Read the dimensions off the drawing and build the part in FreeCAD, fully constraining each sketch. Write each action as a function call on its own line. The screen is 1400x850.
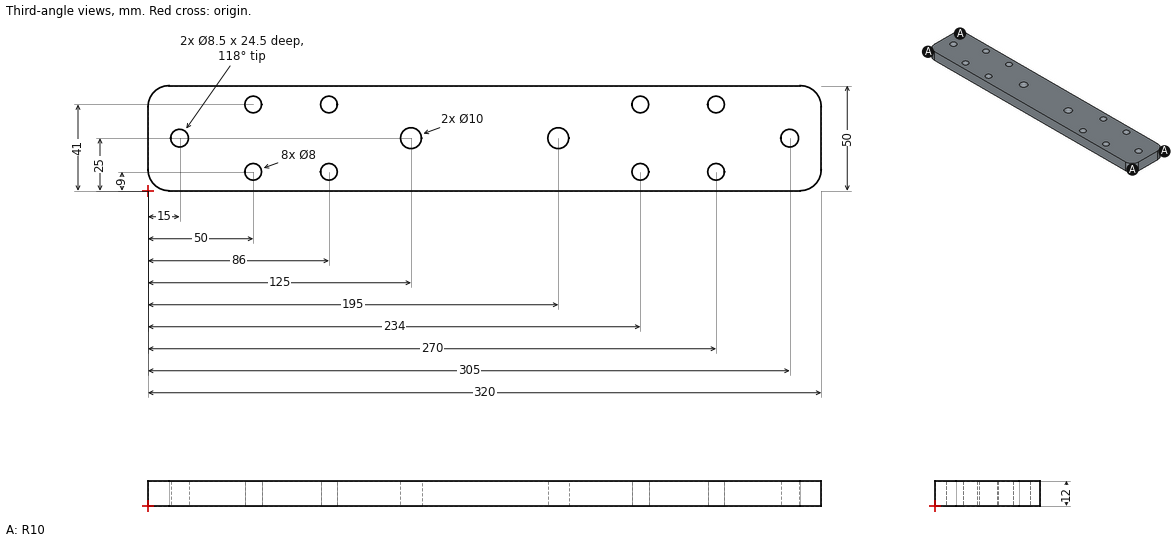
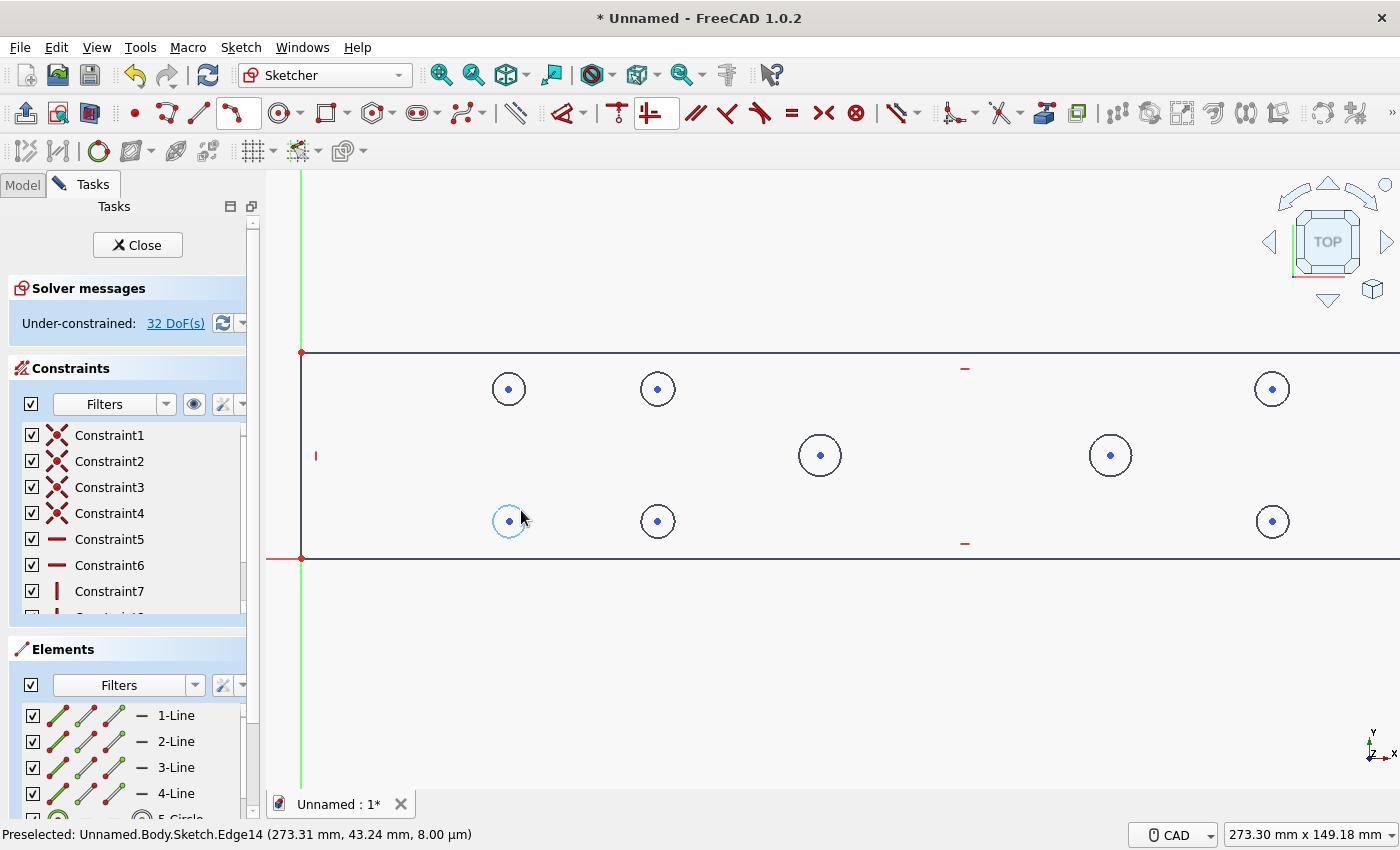
click(521, 510)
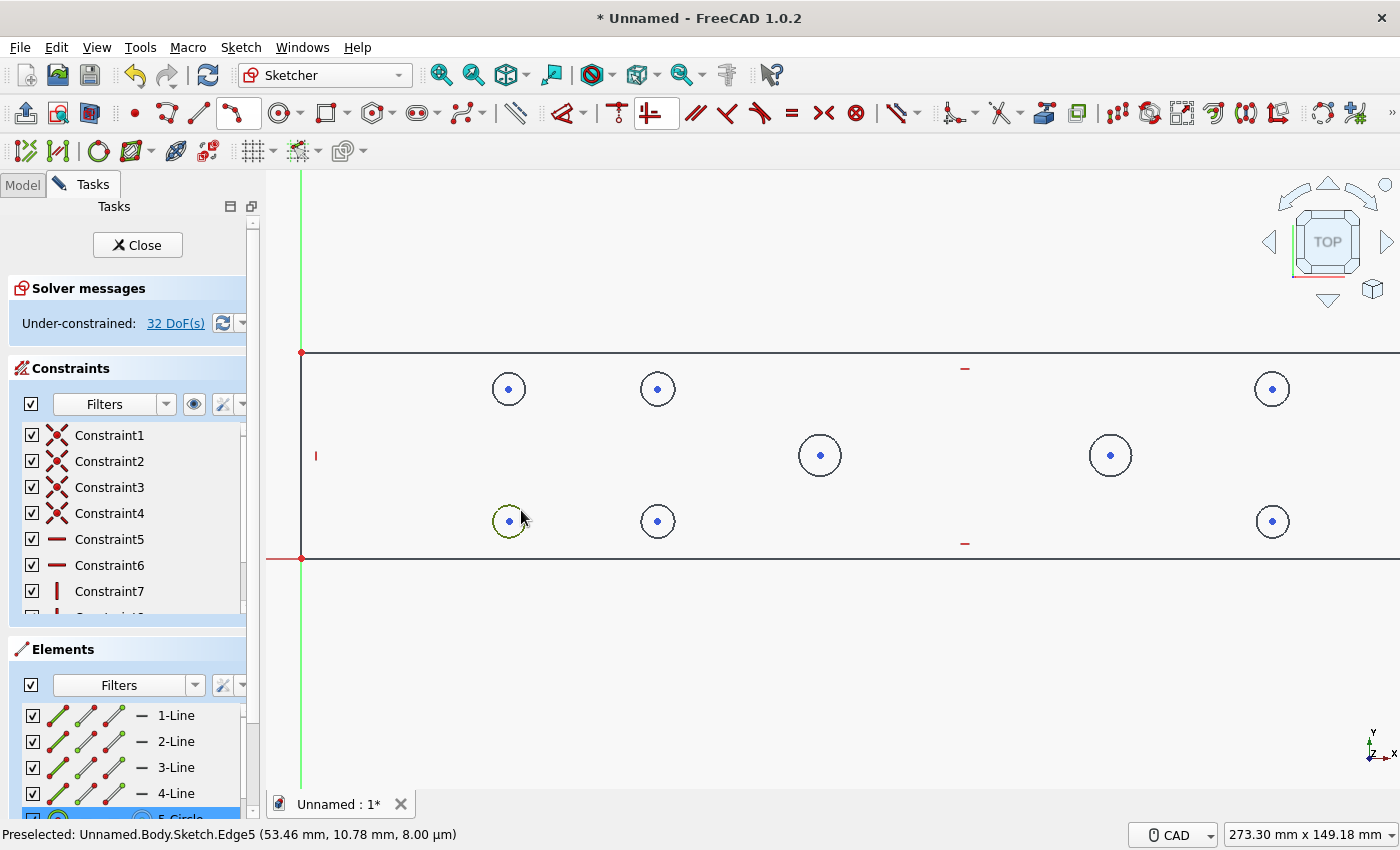
click(670, 510)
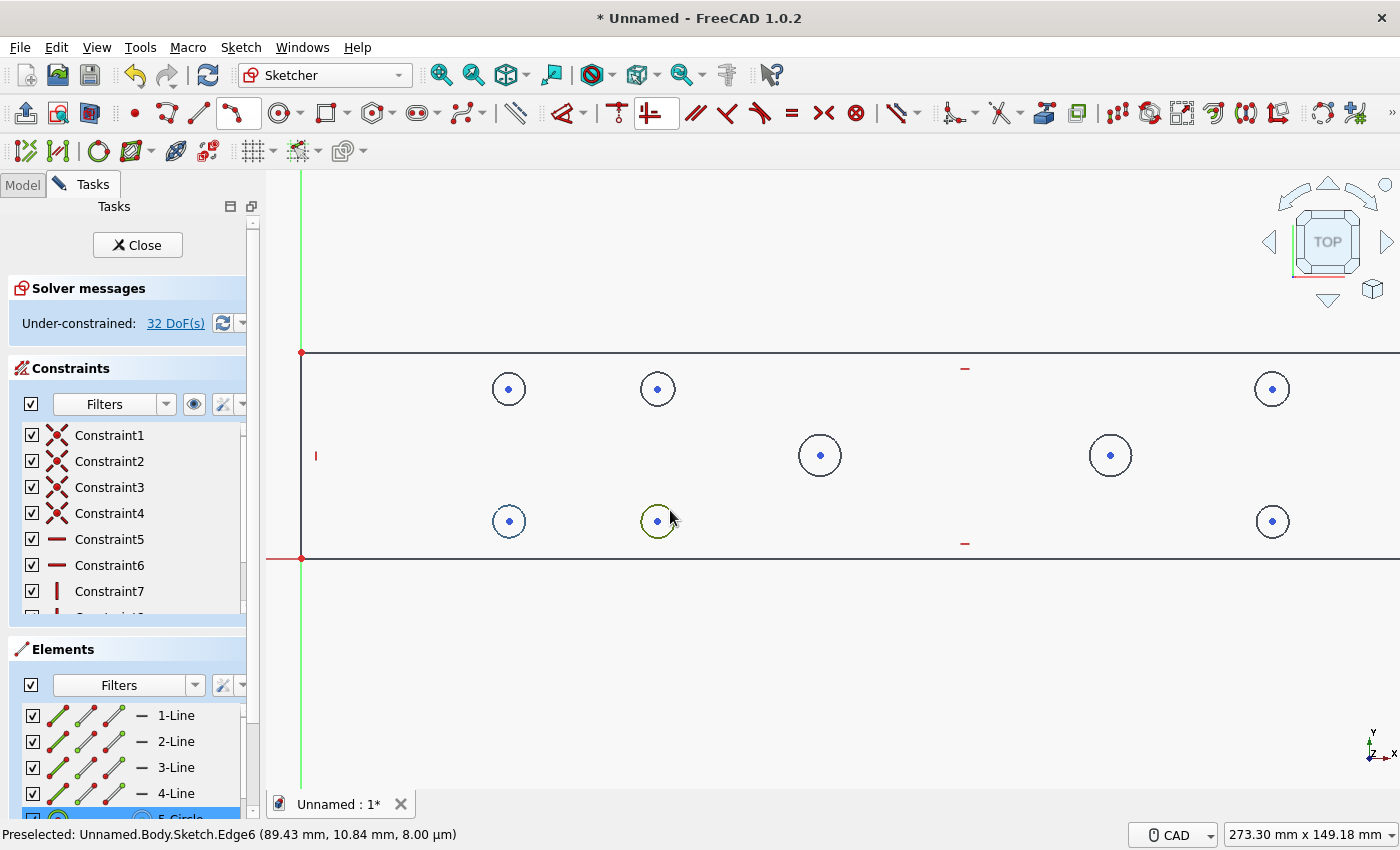
scroll(520, 510, down, 3)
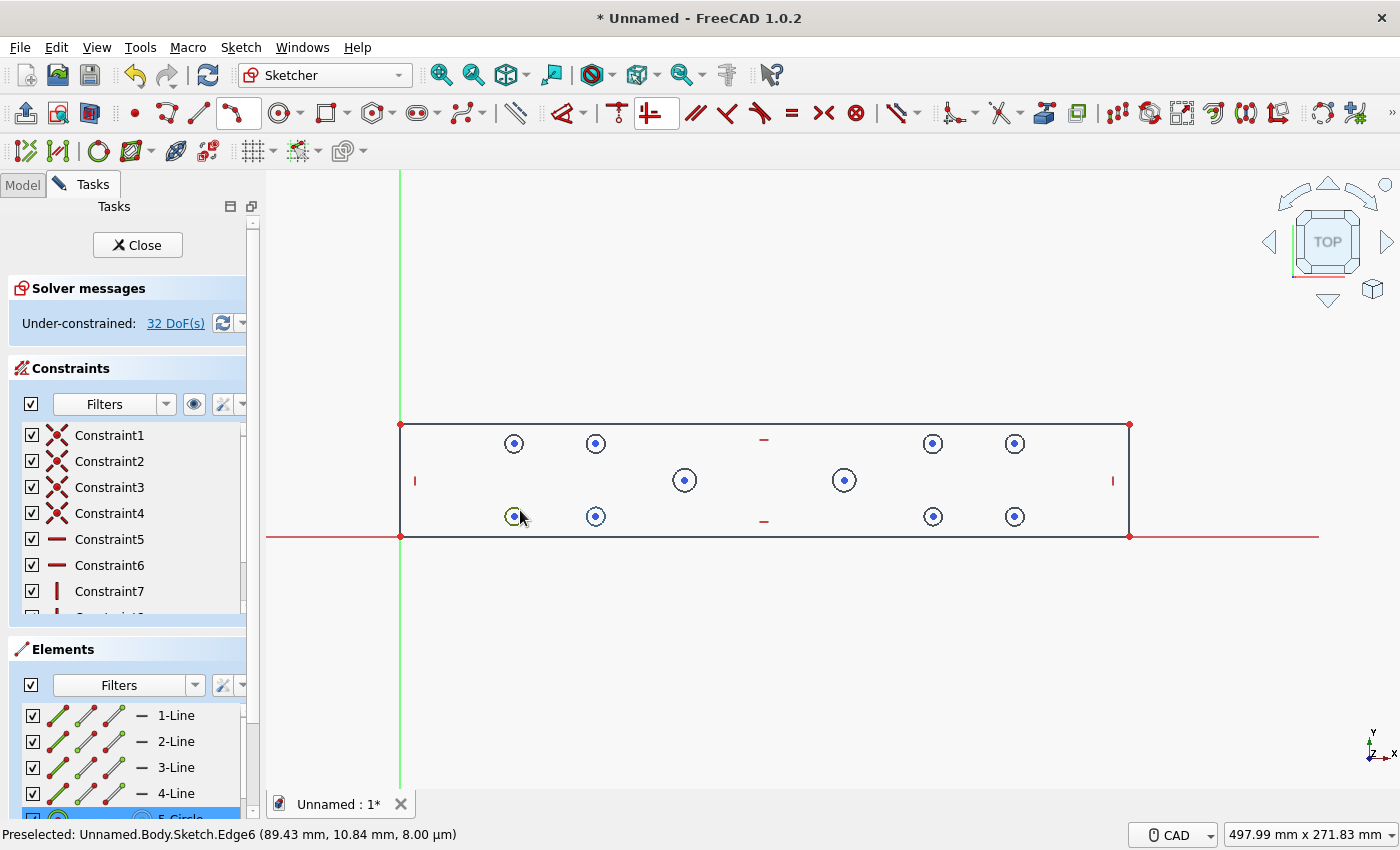
scroll(939, 510, up, 3)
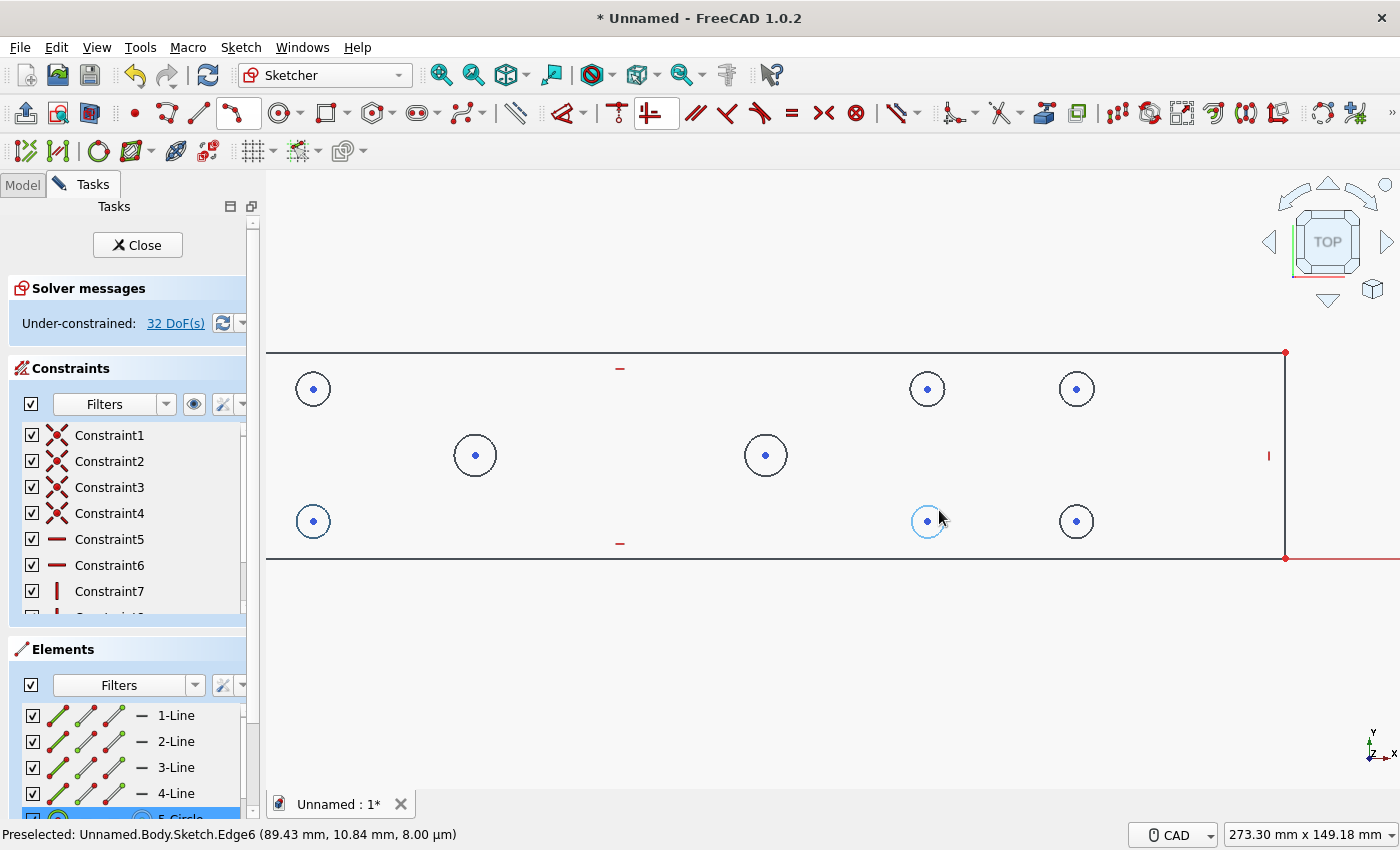
click(939, 510)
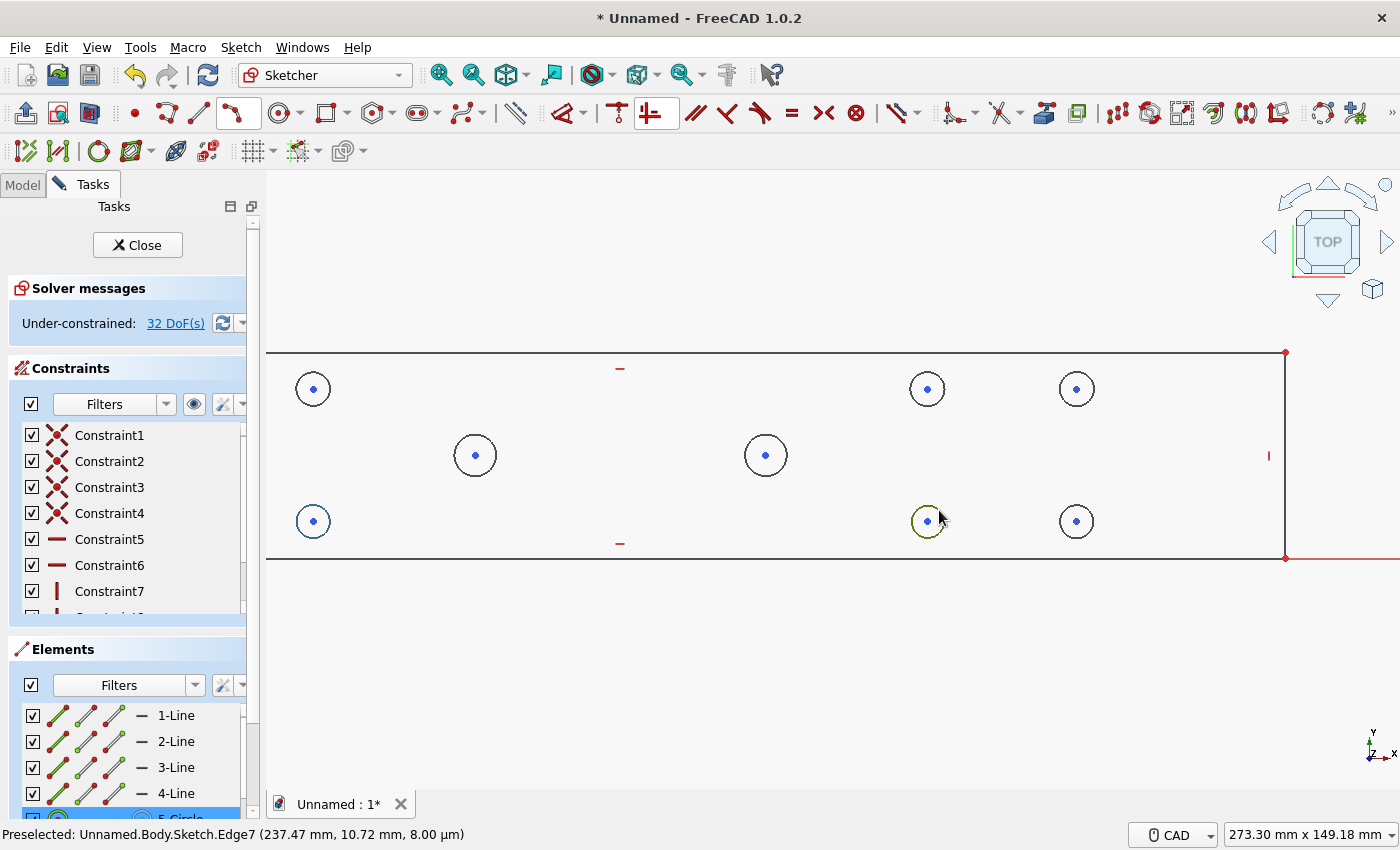
click(1088, 510)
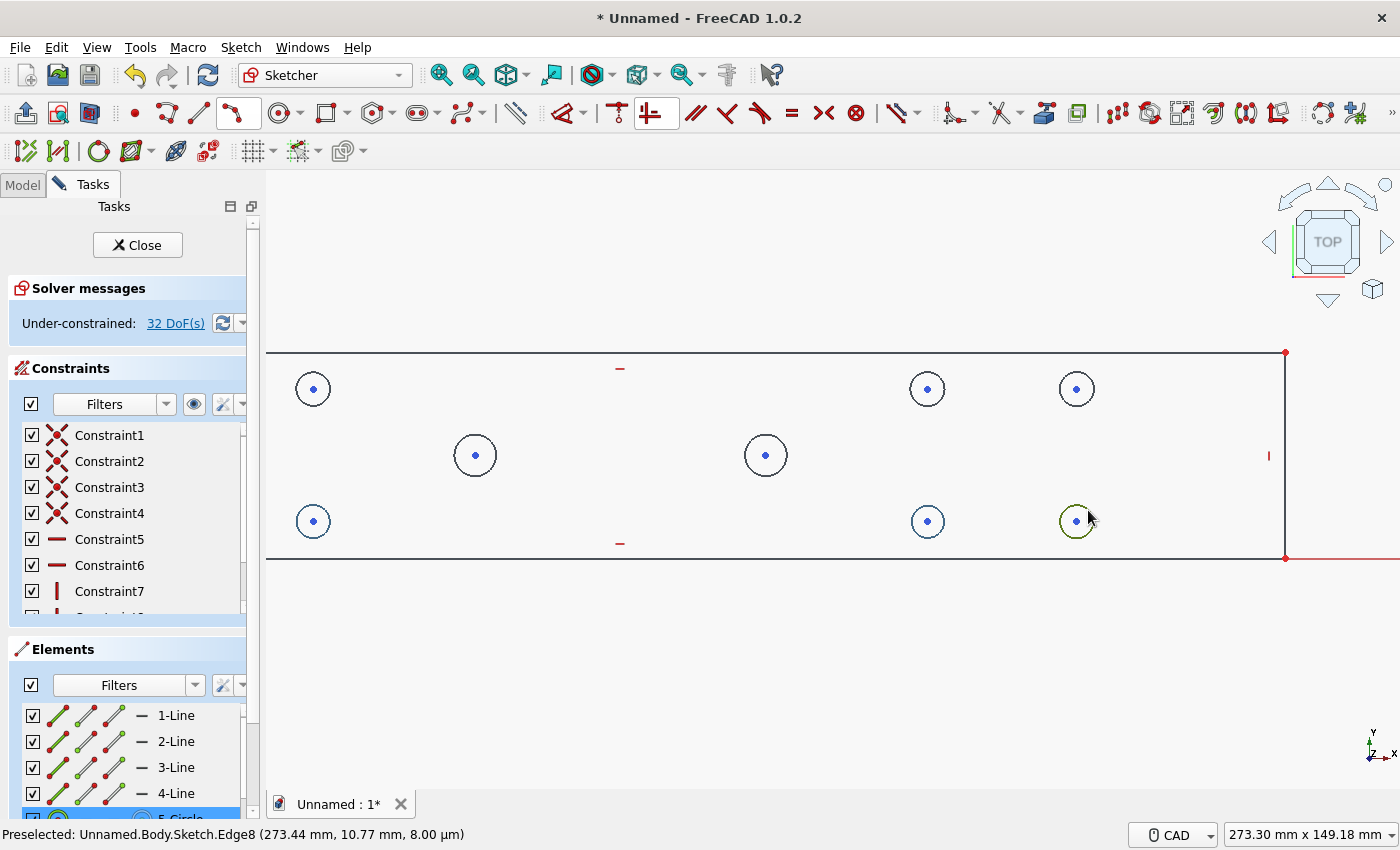
scroll(940, 510, down, 3)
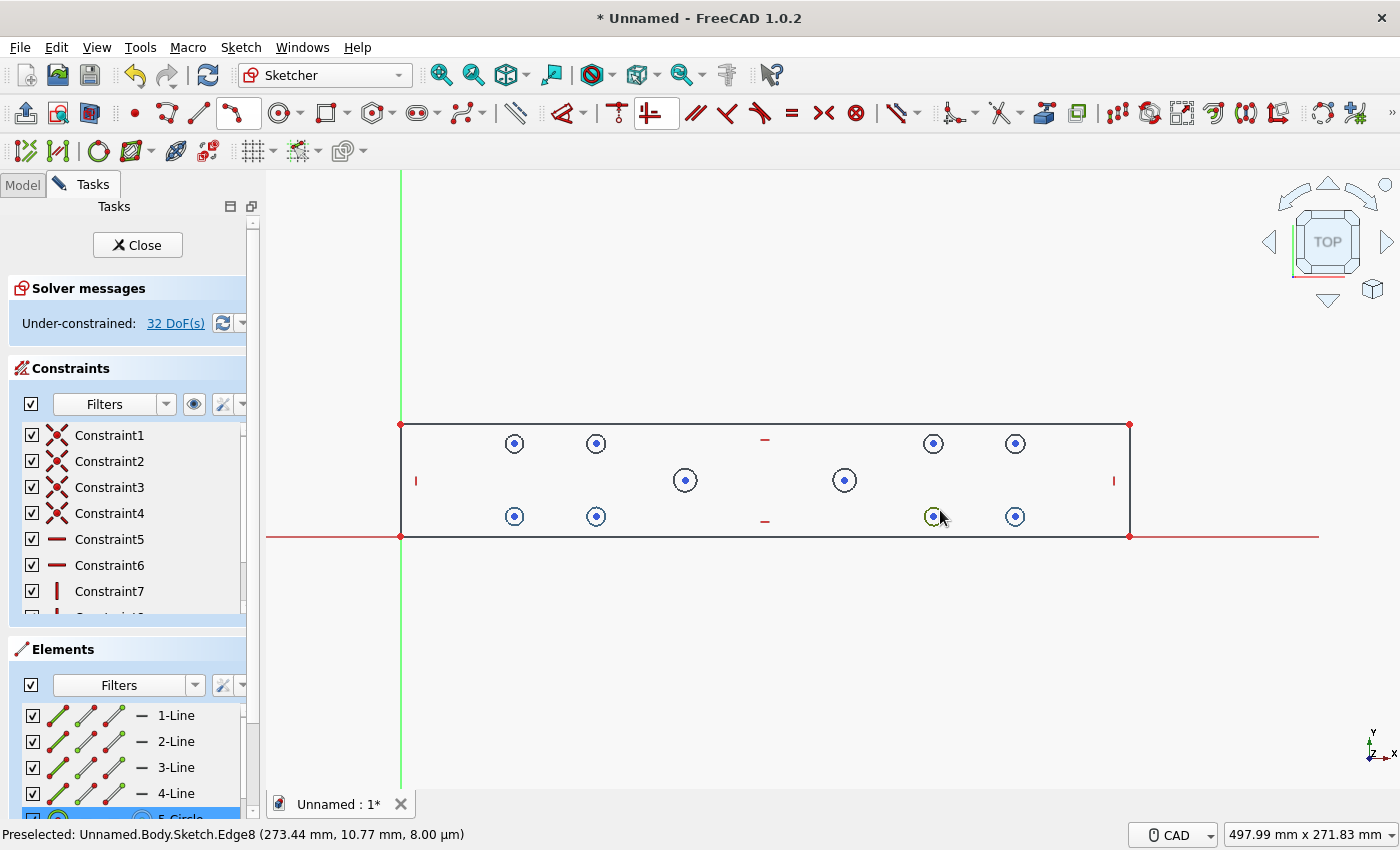
scroll(521, 438, up, 3)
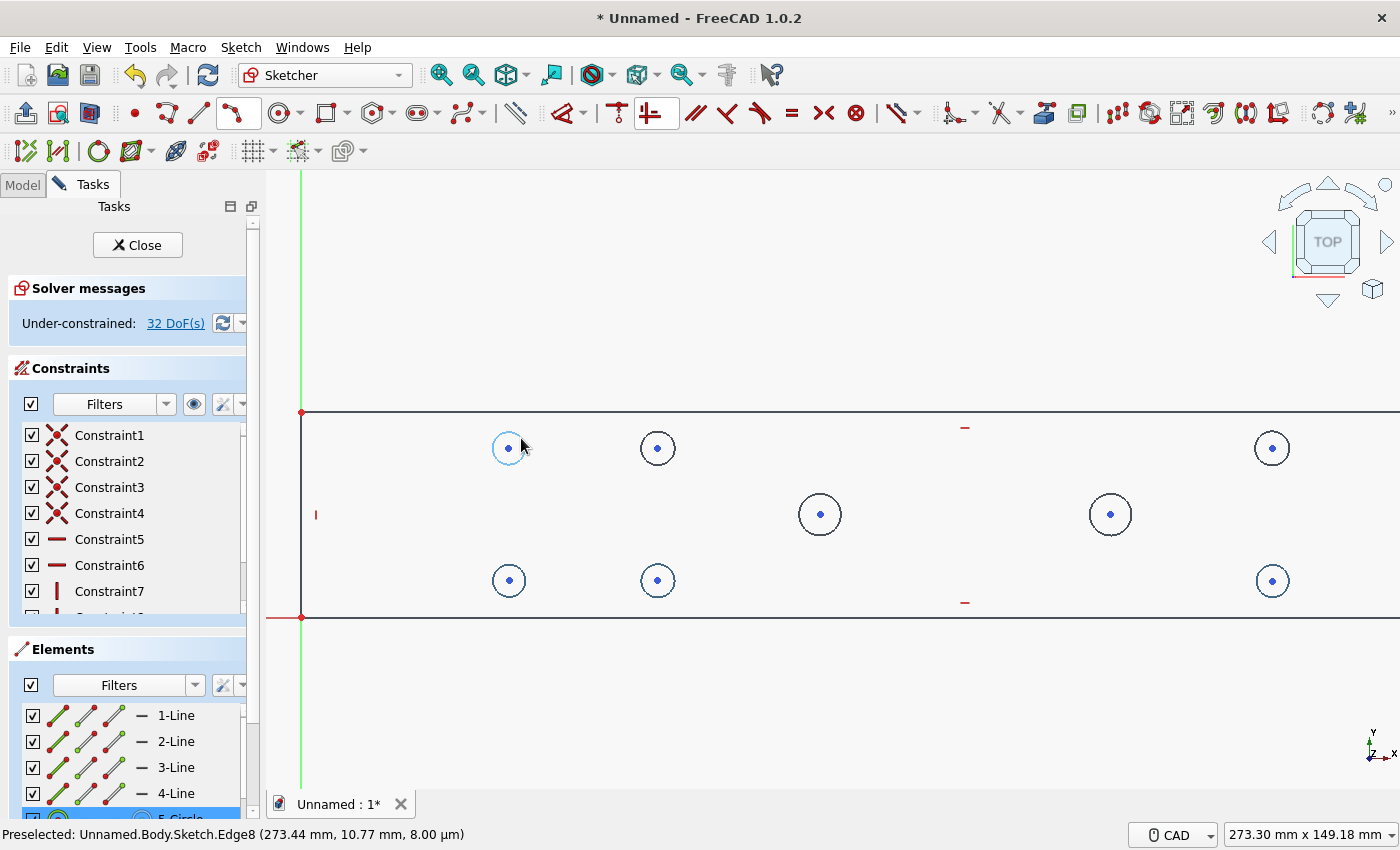
click(520, 437)